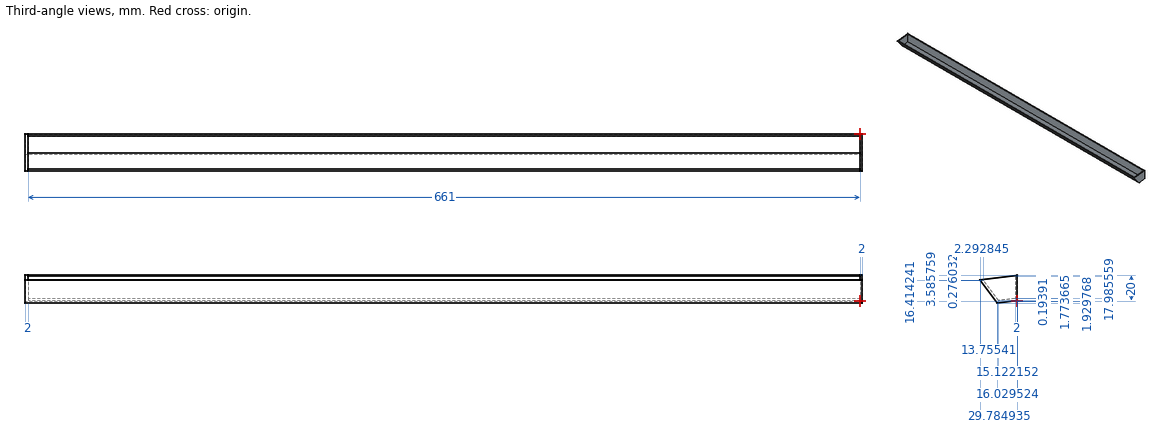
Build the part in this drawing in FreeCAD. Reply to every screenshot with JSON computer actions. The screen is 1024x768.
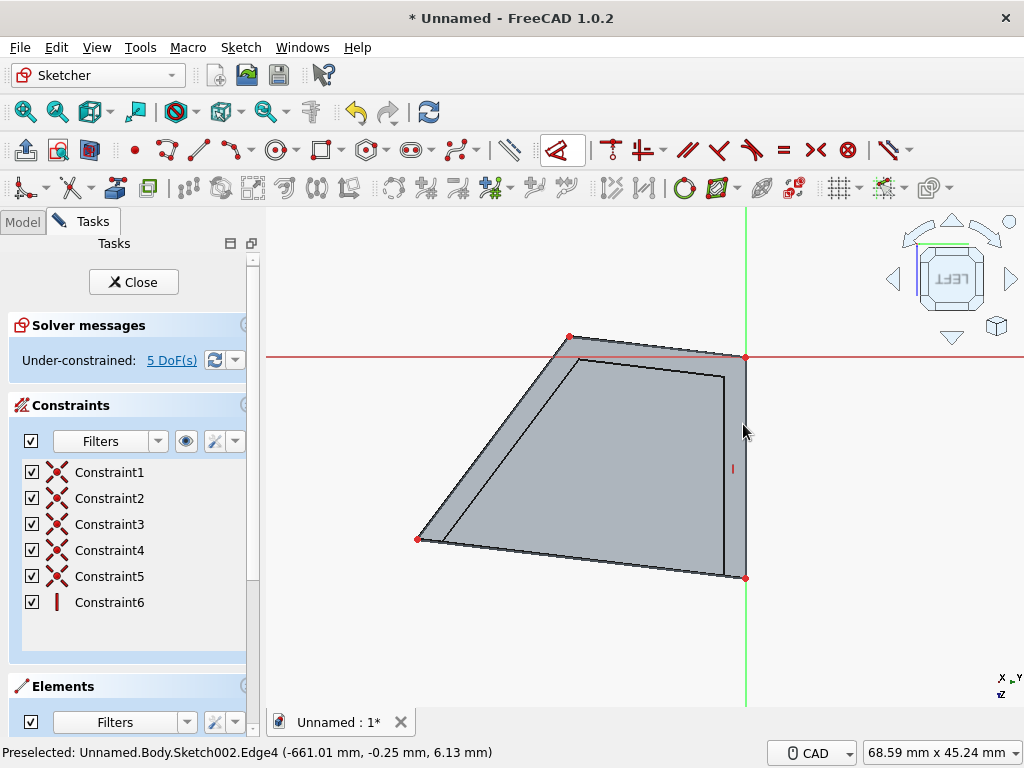
{"action": "left_click", "coordinate": [746, 512]}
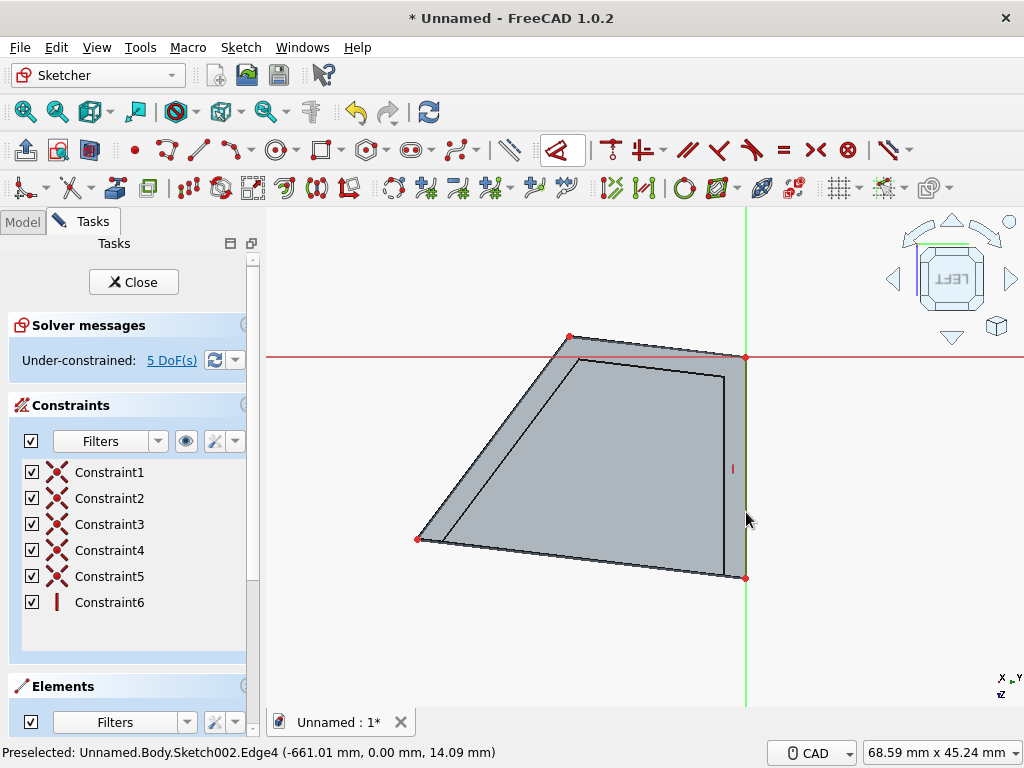
{"action": "key", "text": "i"}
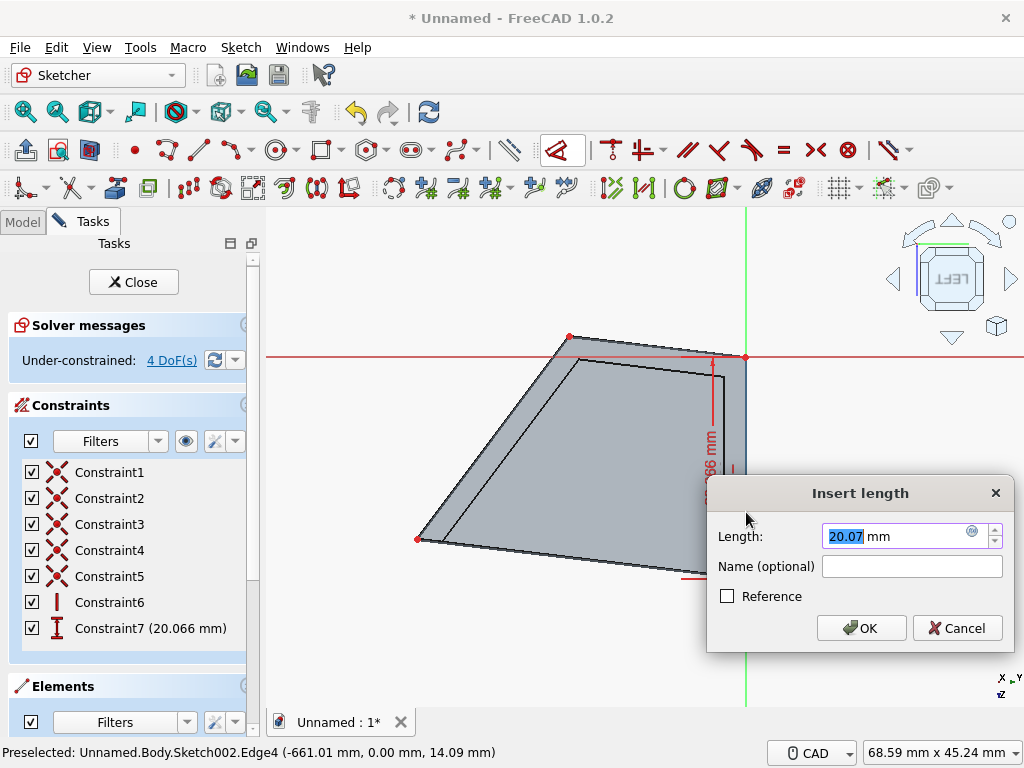
{"action": "type", "text": "20"}
{"action": "key", "text": "Return"}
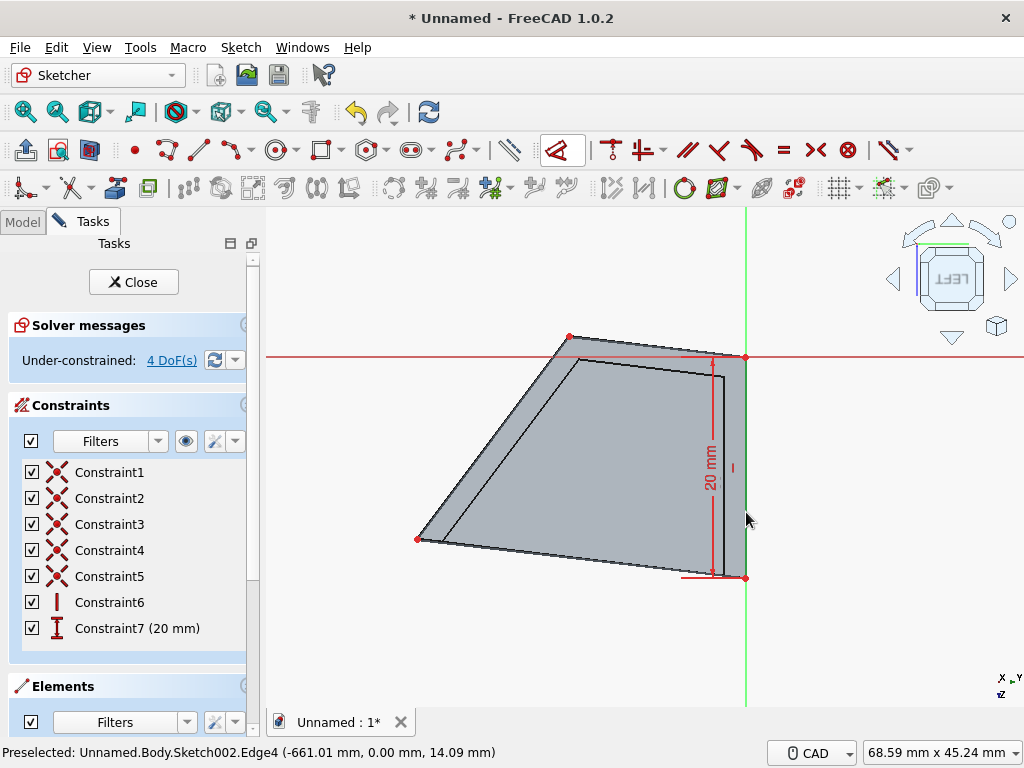
{"action": "scroll", "coordinate": [569, 337], "scroll_direction": "up", "scroll_amount": 4}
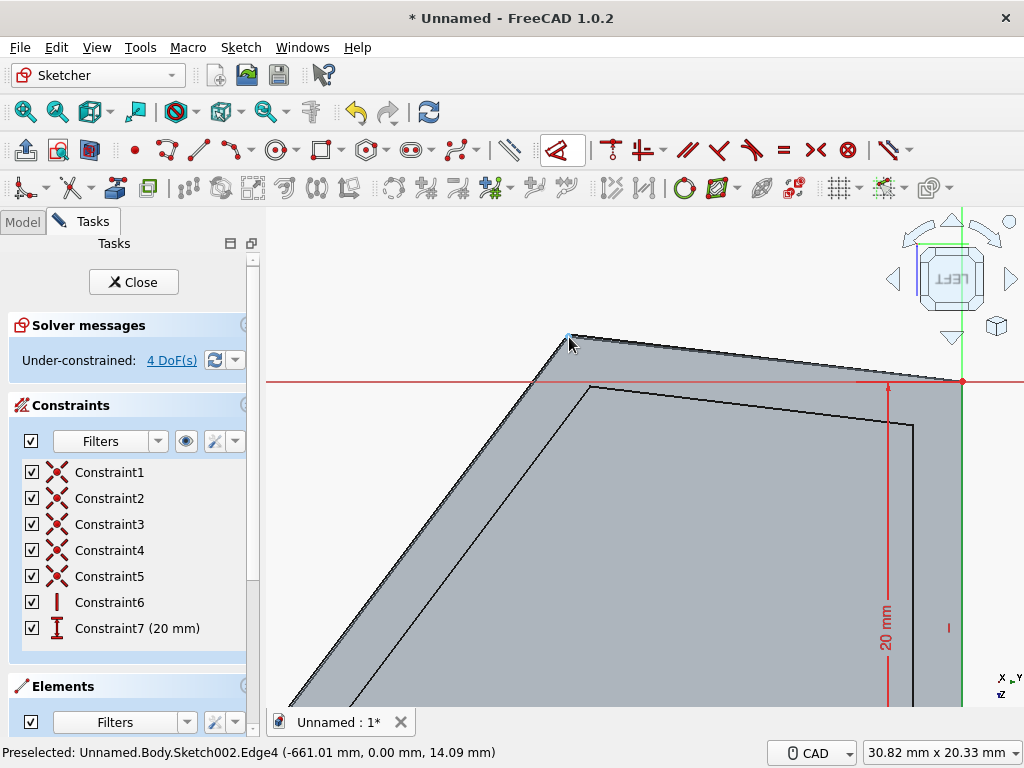
{"action": "left_click", "coordinate": [569, 337]}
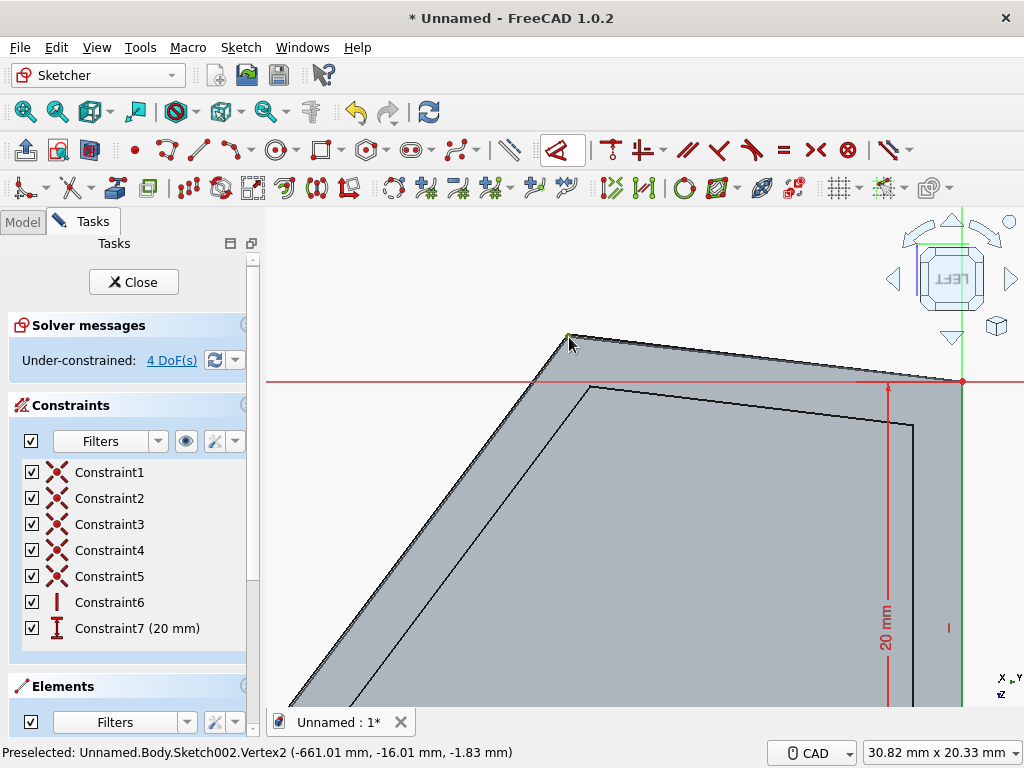
{"action": "key", "text": "i"}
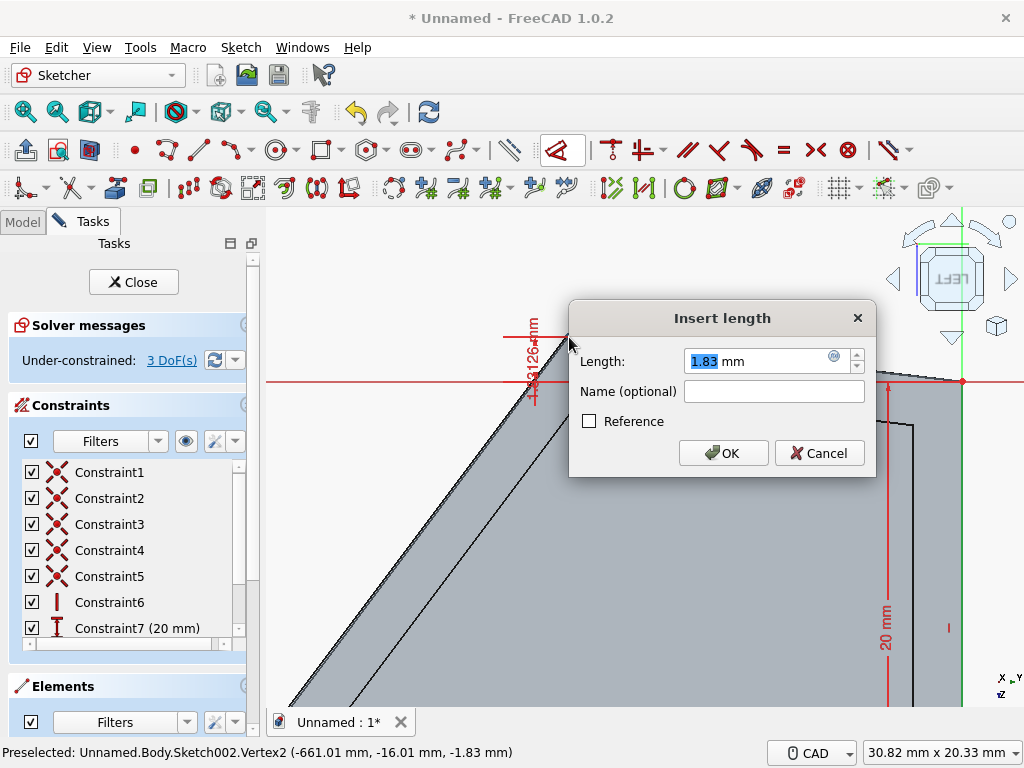
{"action": "type", "text": "1.929768"}
{"action": "key", "text": "Return"}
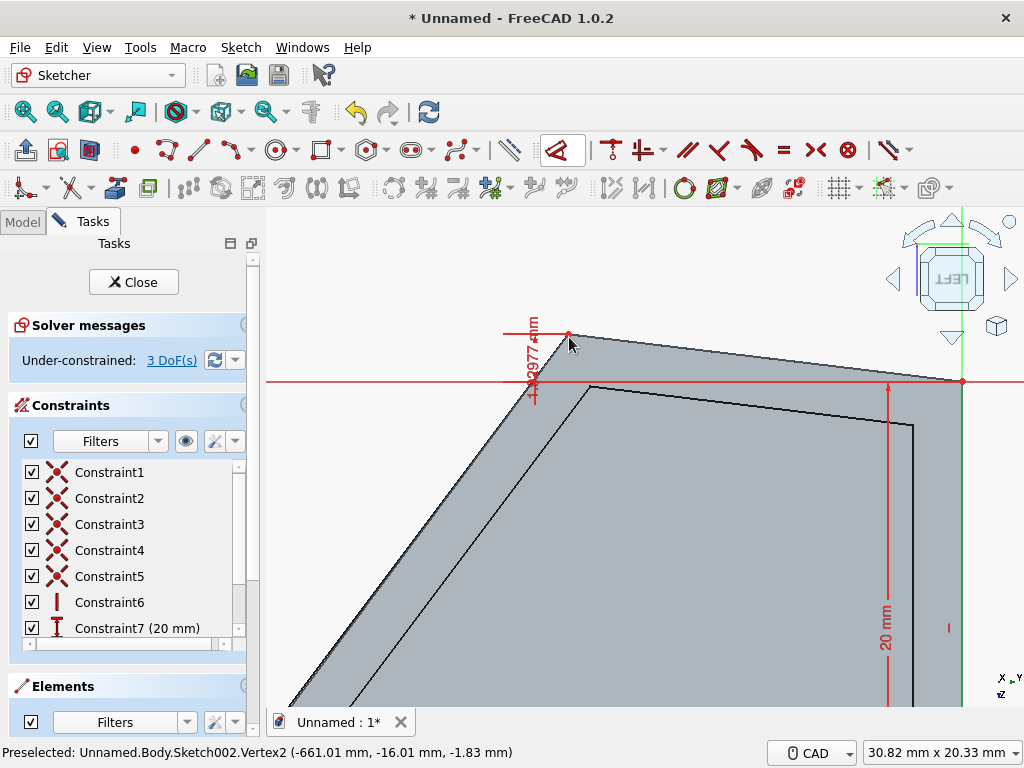
{"action": "left_click", "coordinate": [467, 471]}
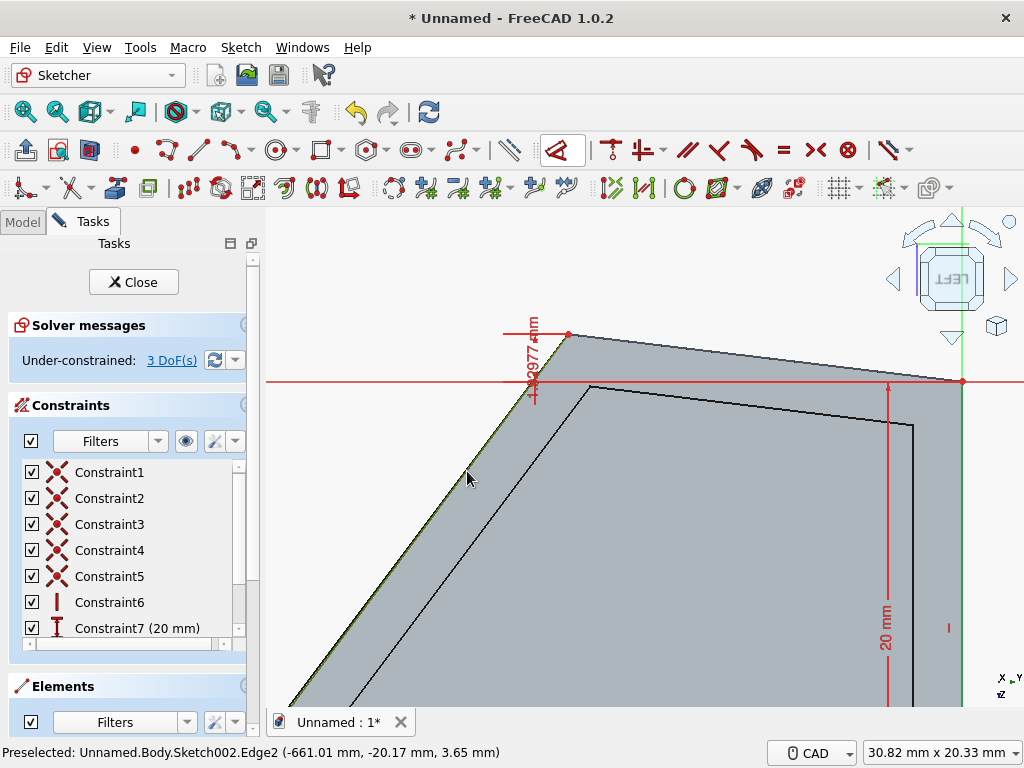
{"action": "key", "text": "l"}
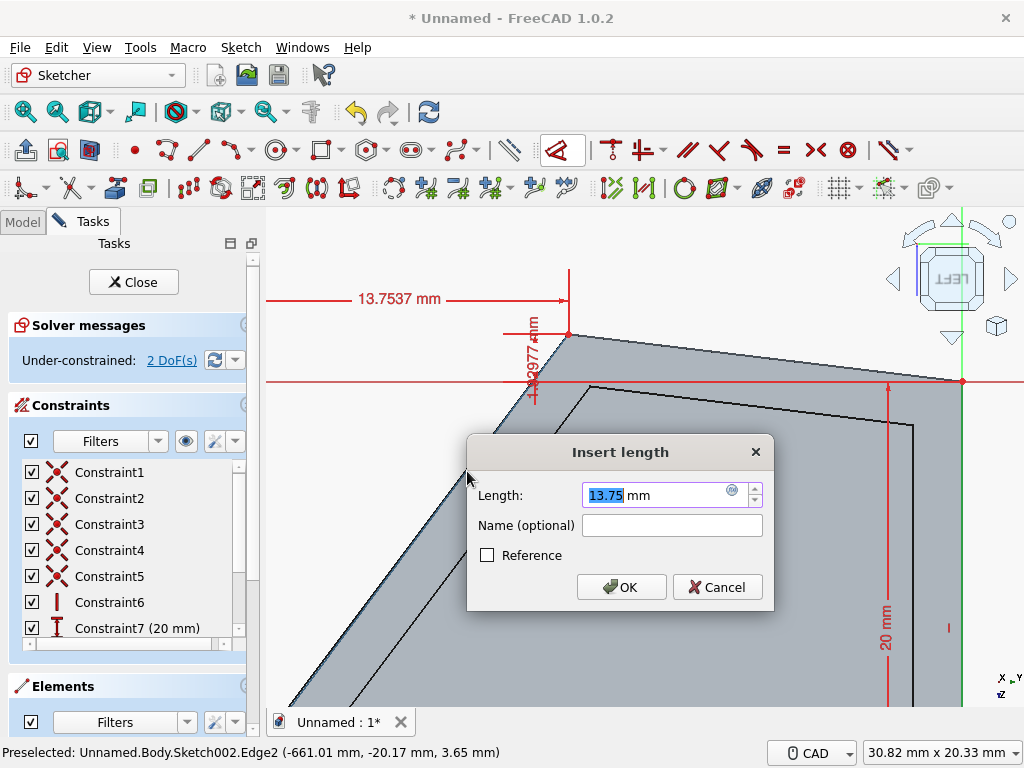
{"action": "type", "text": "13.75541"}
{"action": "key", "text": "Return"}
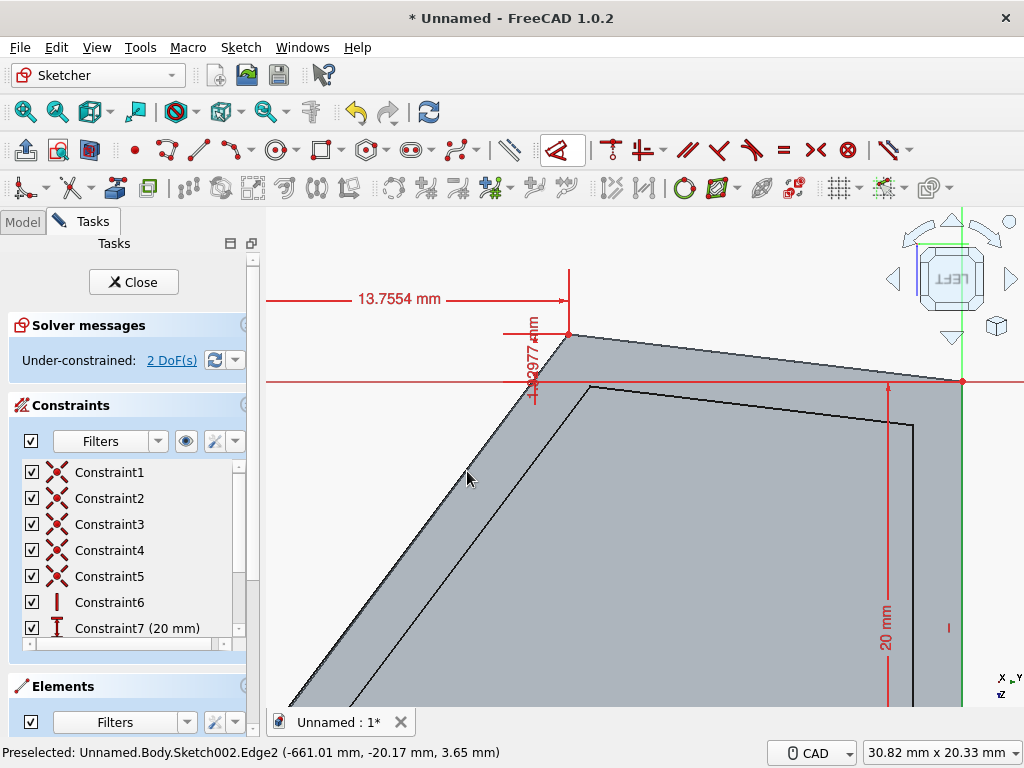
{"action": "scroll", "coordinate": [553, 278], "scroll_direction": "down", "scroll_amount": 3}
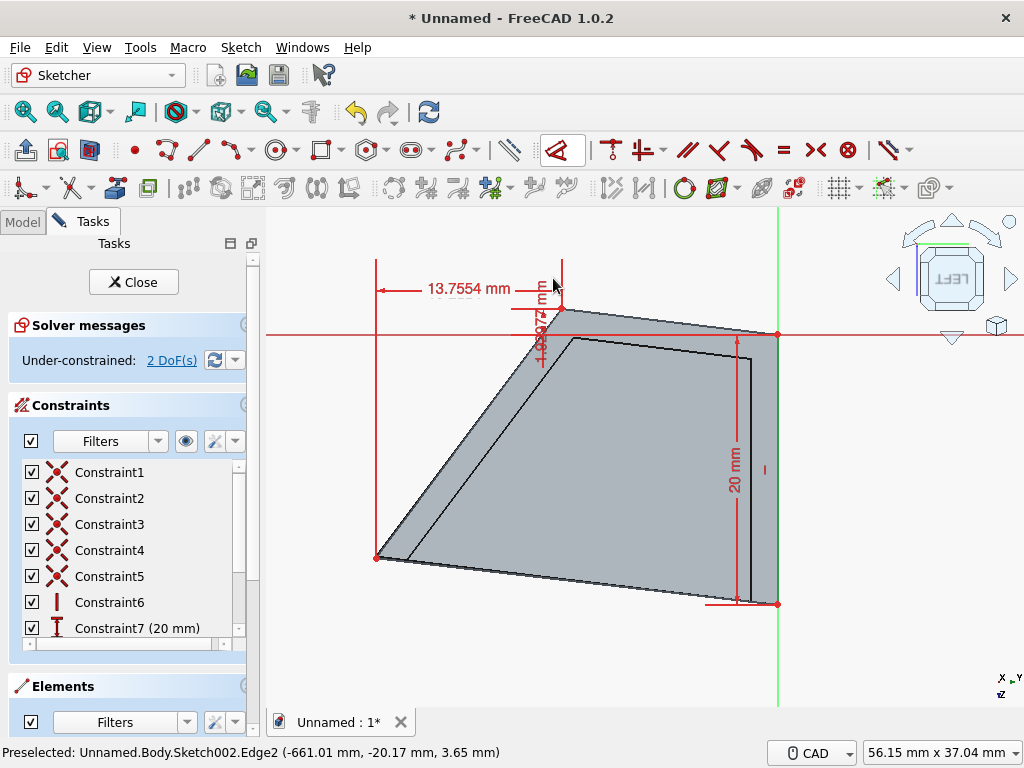
{"action": "left_click", "coordinate": [497, 572]}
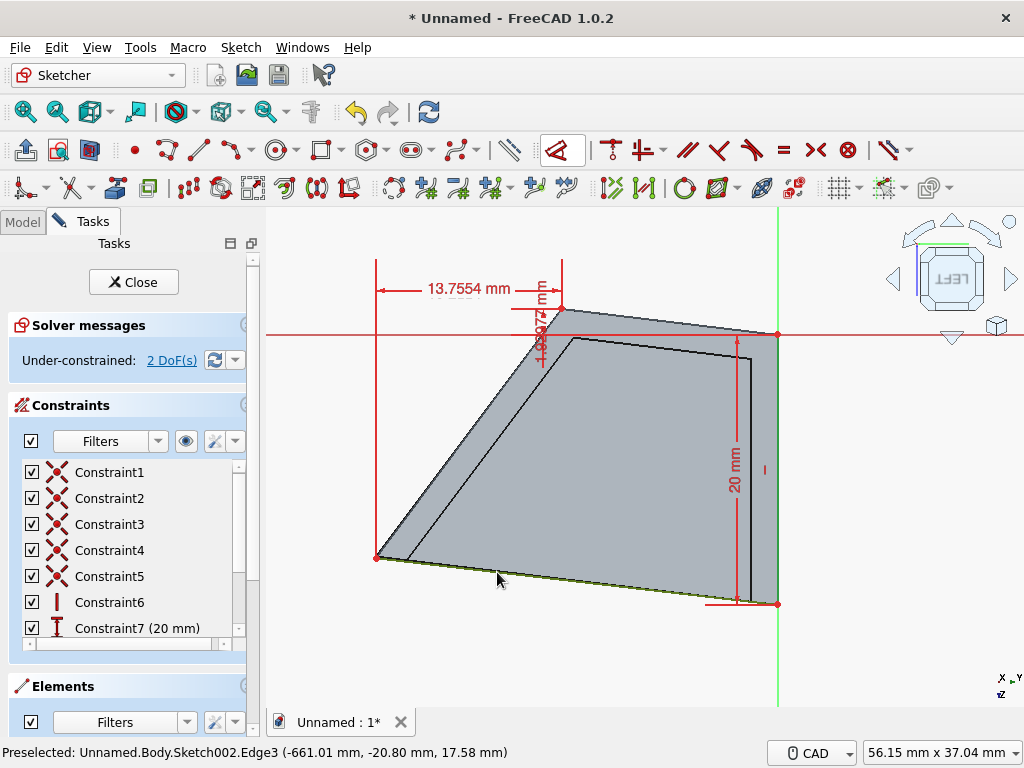
{"action": "key", "text": "i"}